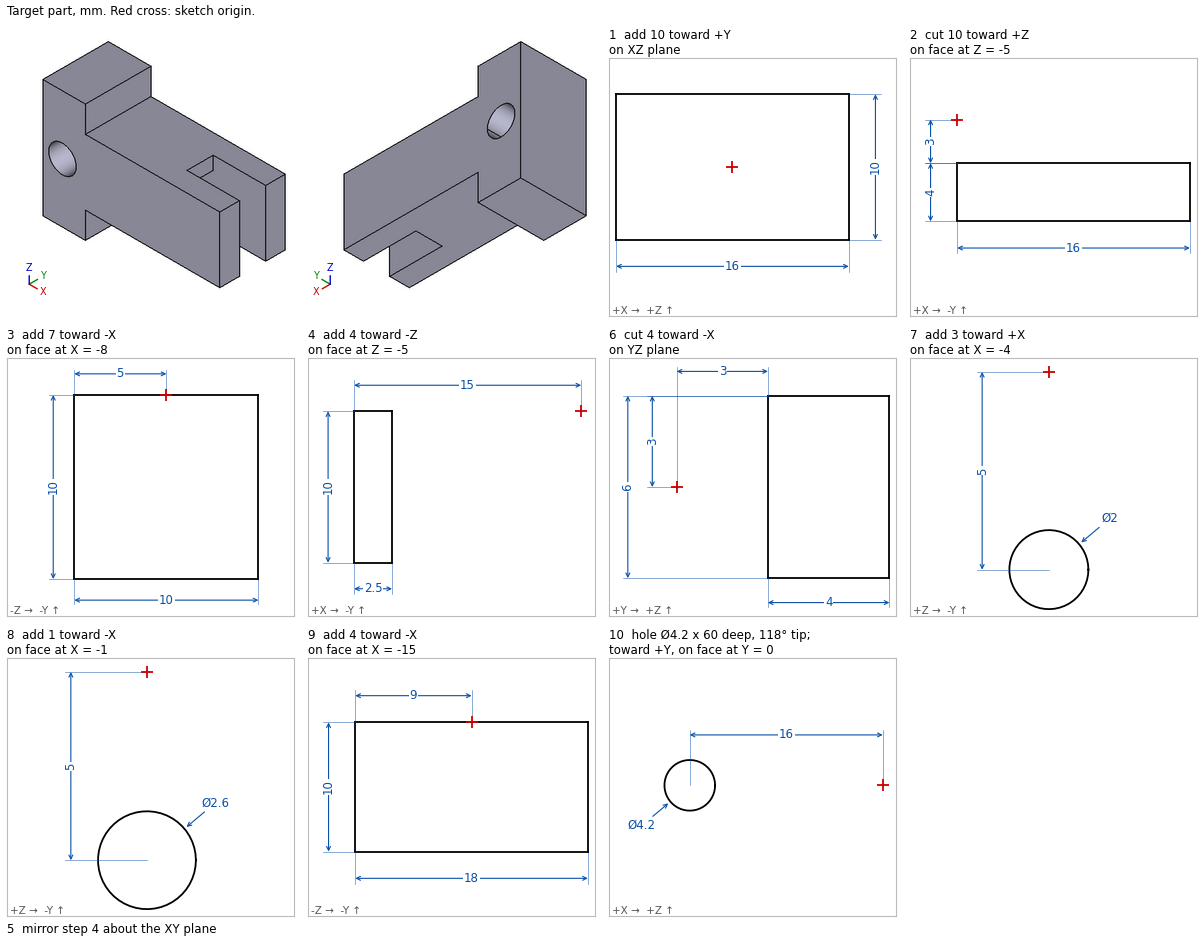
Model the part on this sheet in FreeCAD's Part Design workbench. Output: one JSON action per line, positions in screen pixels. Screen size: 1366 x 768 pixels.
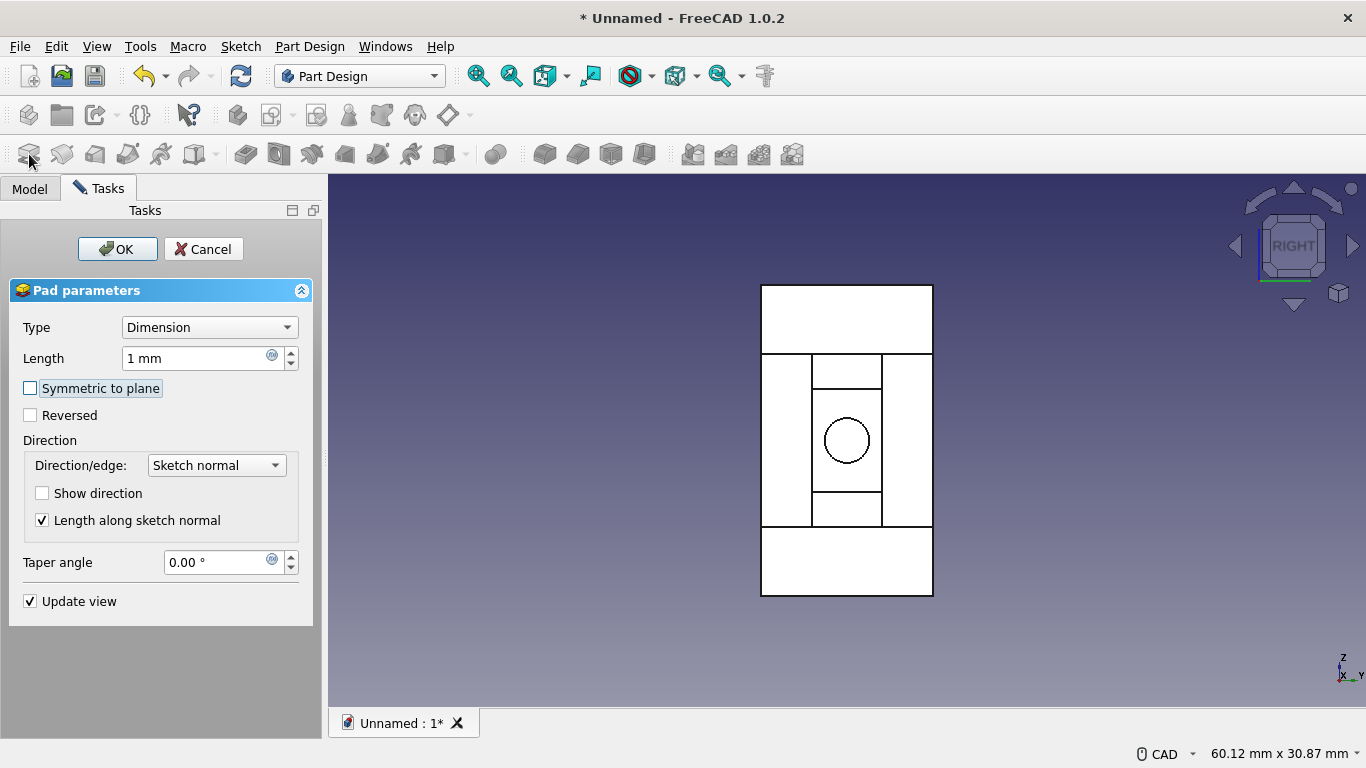
{"action": "left_click", "coordinate": [31, 415]}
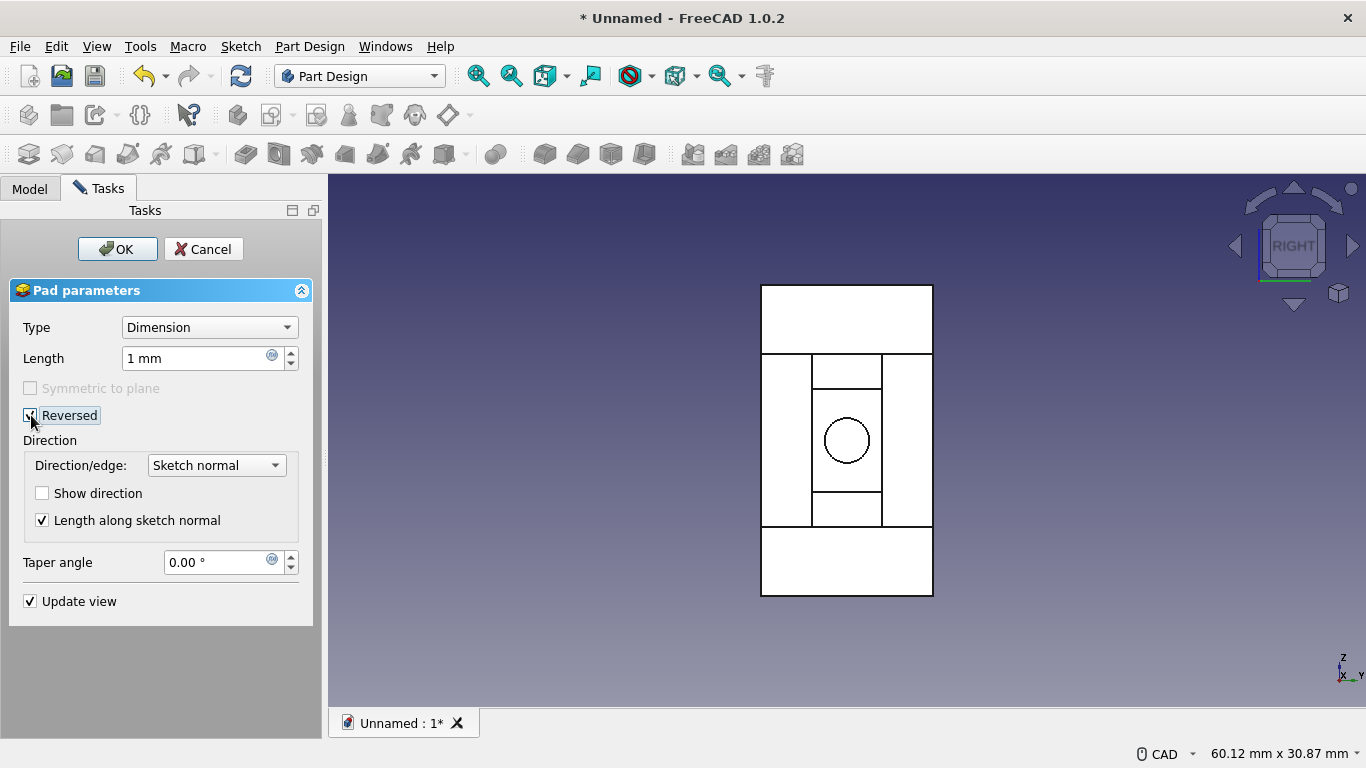
{"action": "left_click", "coordinate": [118, 249]}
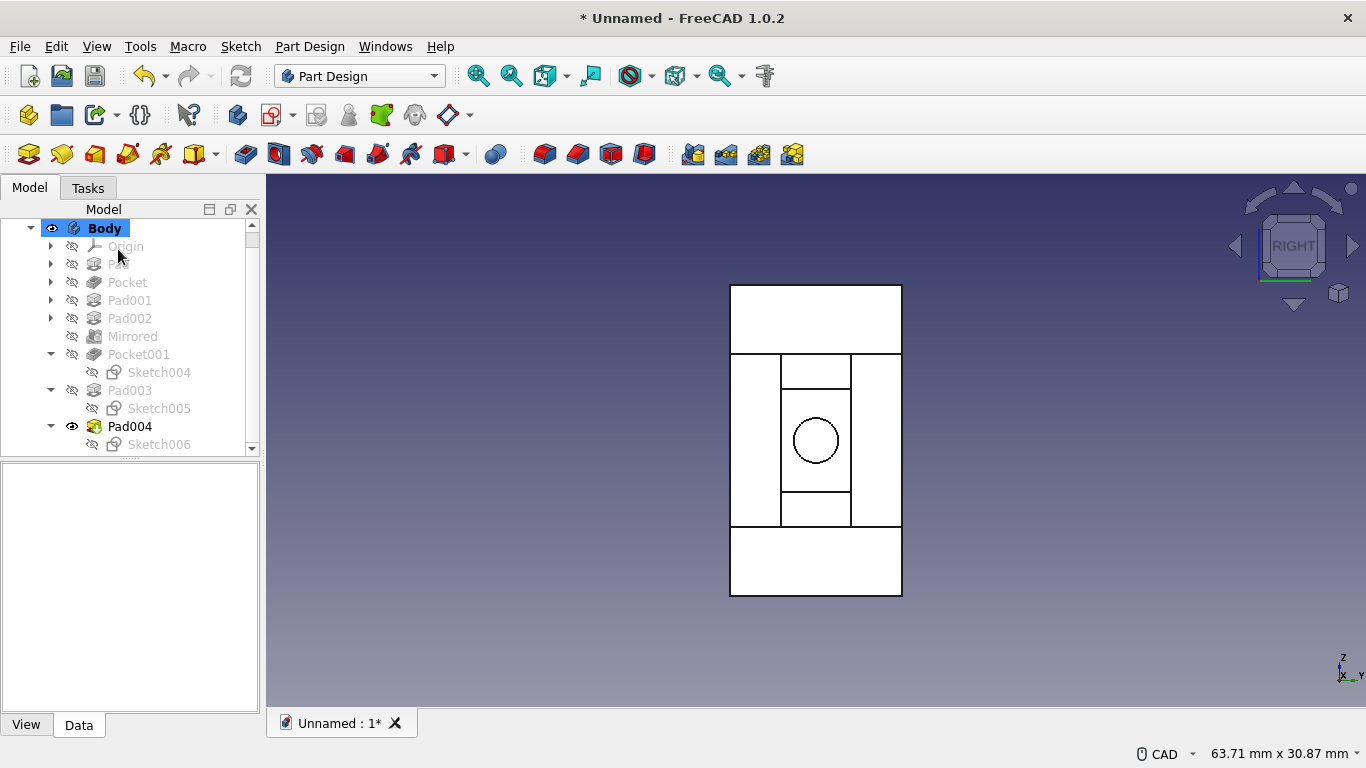
{"action": "key", "text": "6"}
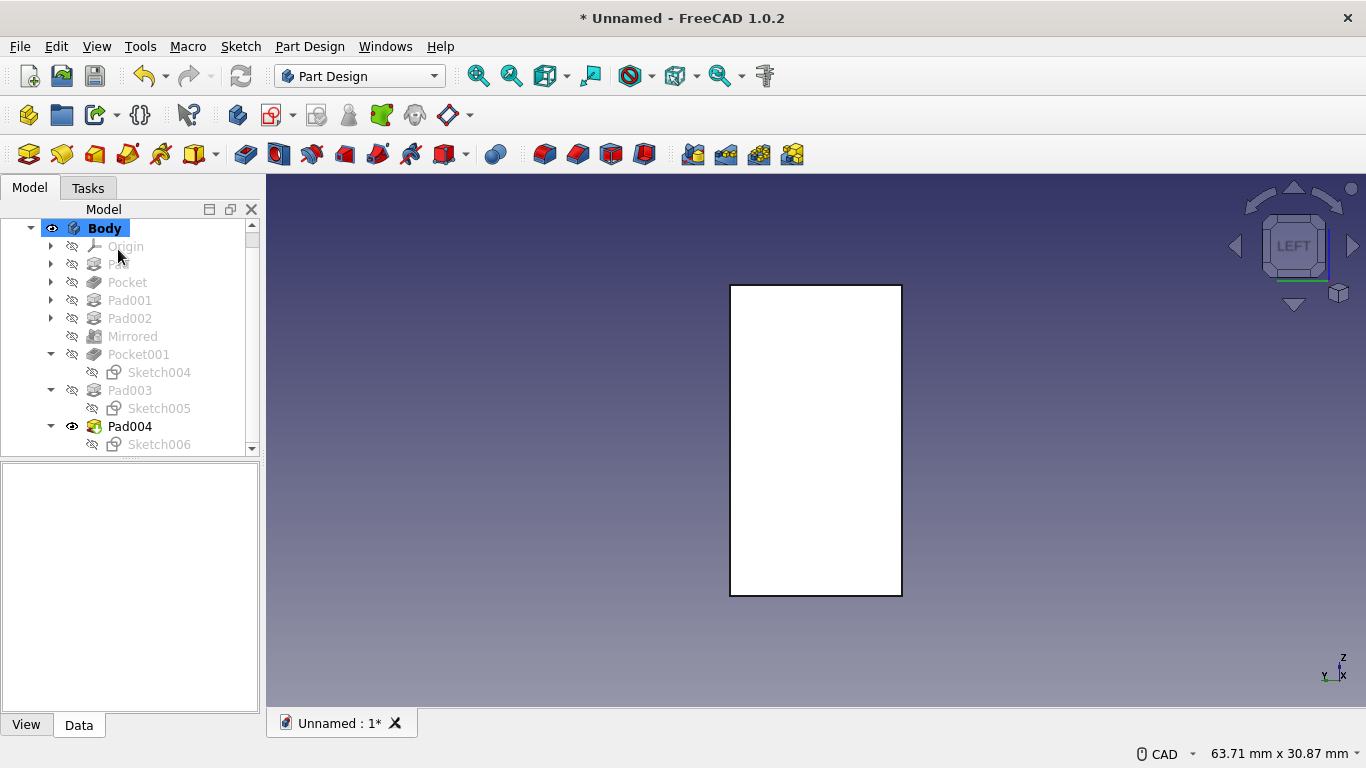
{"action": "left_click", "coordinate": [816, 395]}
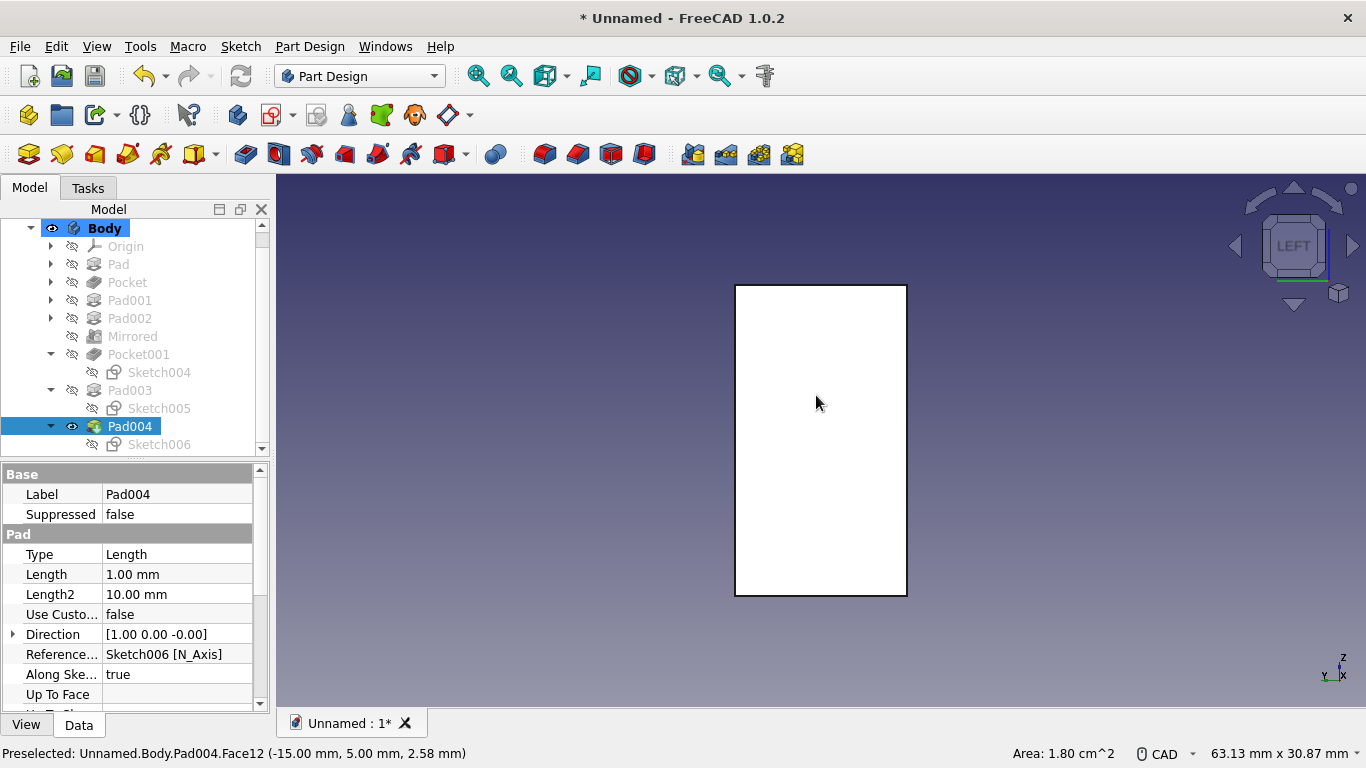
{"action": "left_click", "coordinate": [270, 116]}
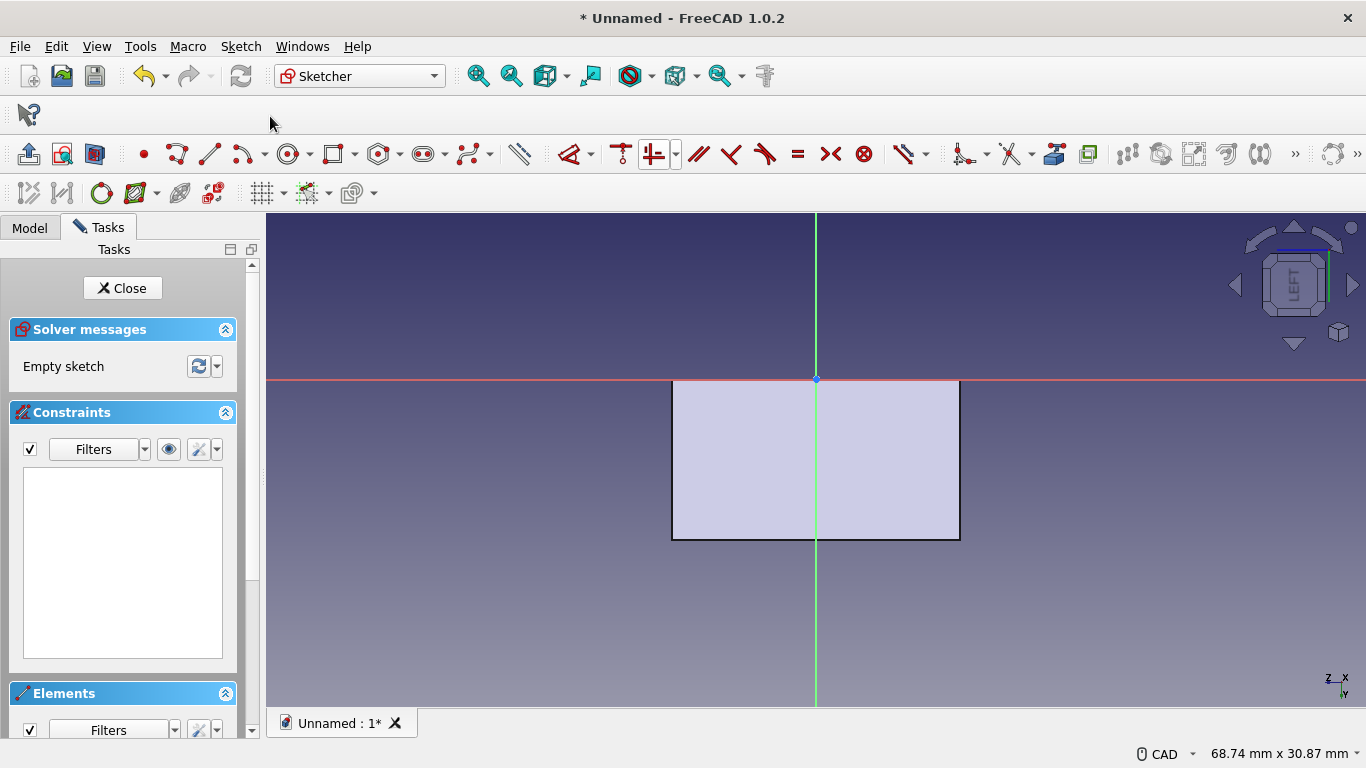
{"action": "scroll", "coordinate": [899, 460], "scroll_direction": "up", "scroll_amount": 3}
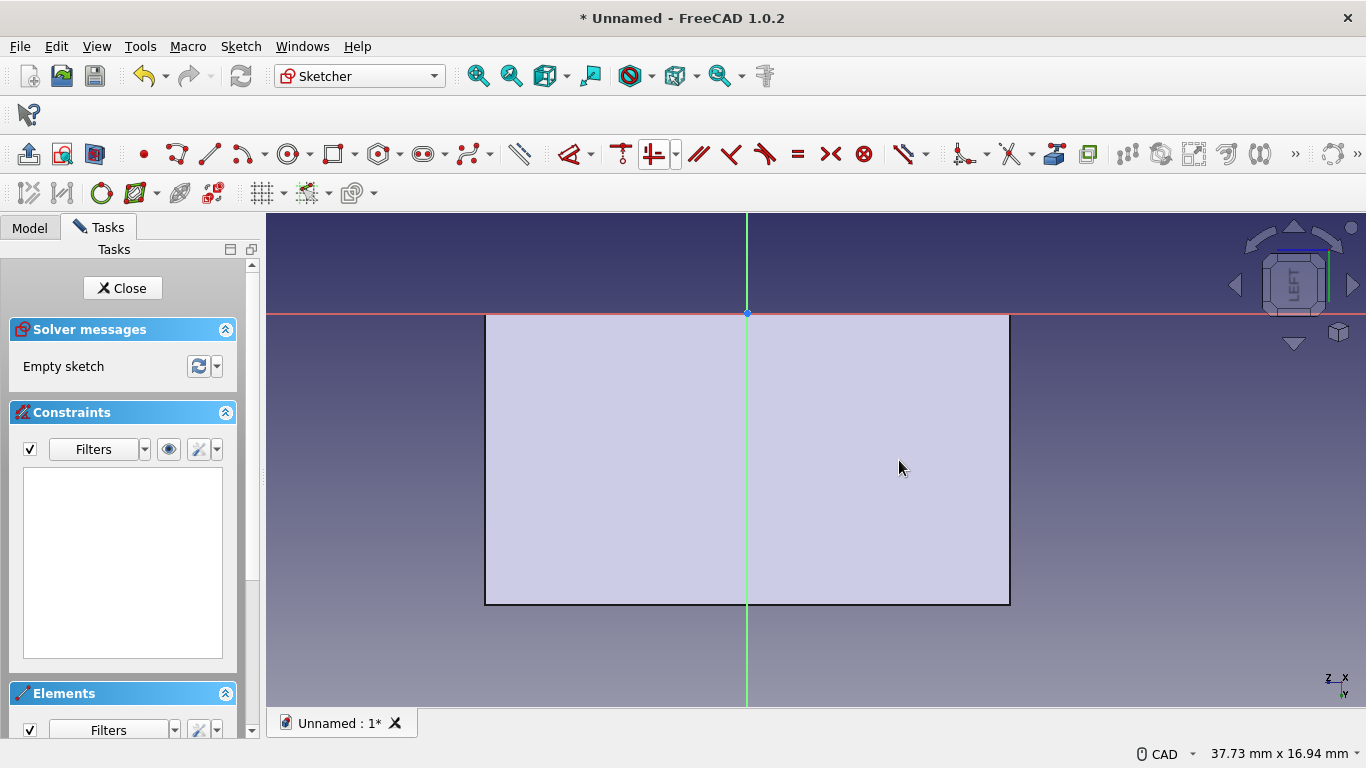
{"action": "left_click", "coordinate": [332, 154]}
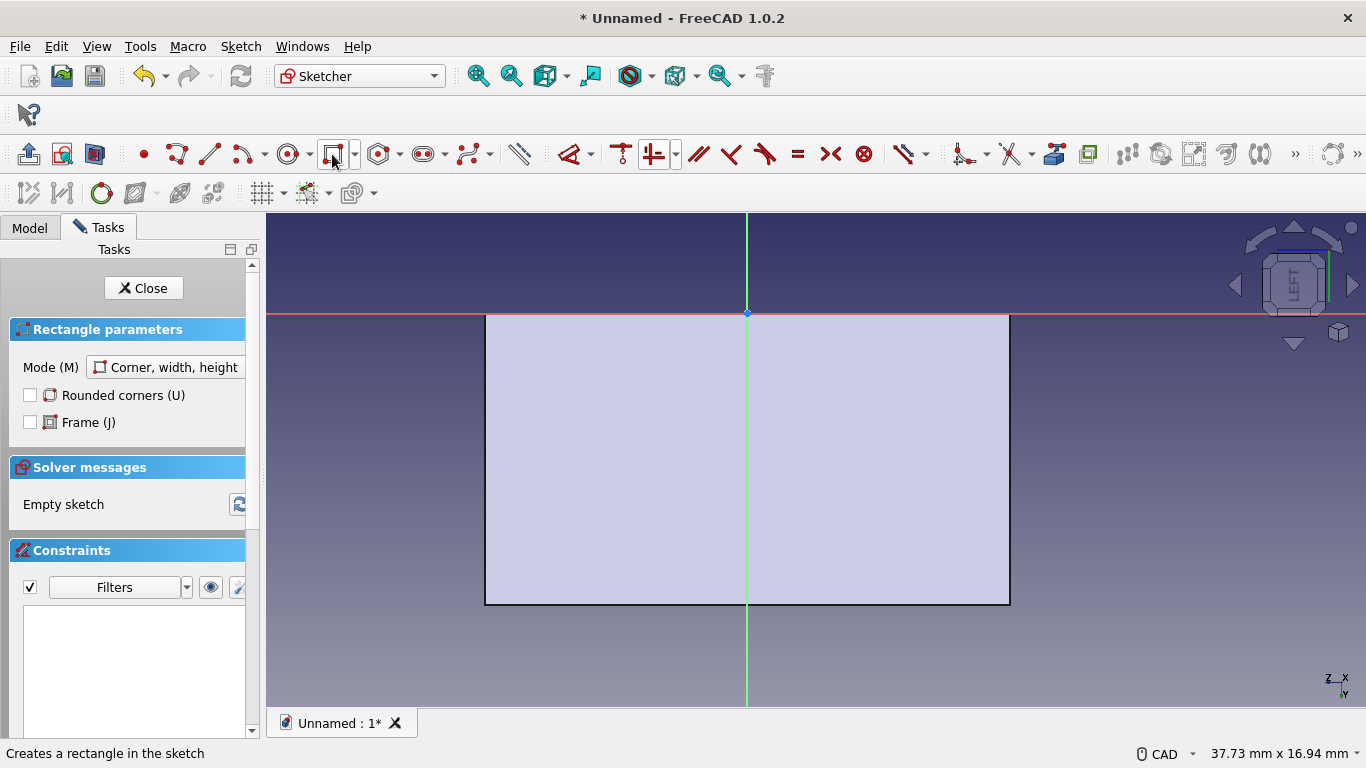
{"action": "left_click", "coordinate": [485, 314]}
{"action": "left_click", "coordinate": [1010, 605]}
{"action": "key", "text": "Escape"}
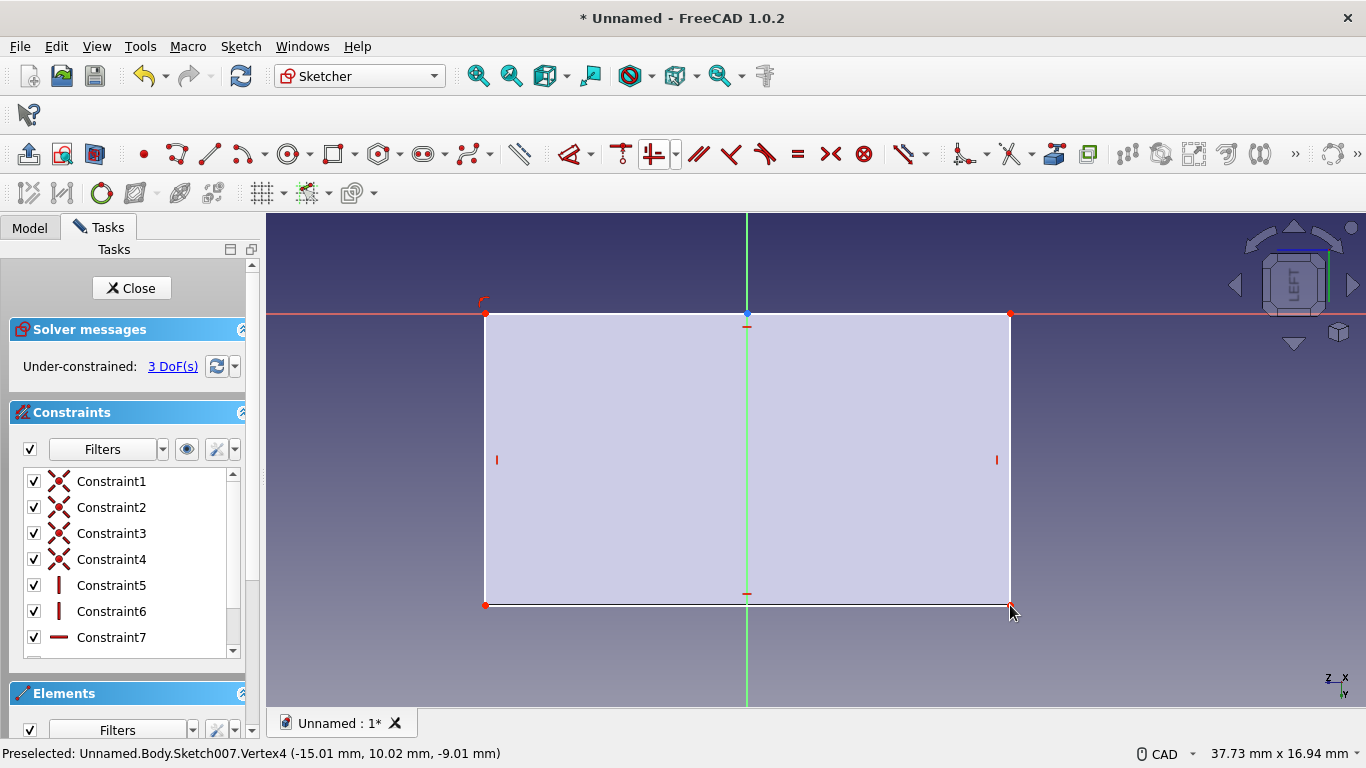
{"action": "left_click", "coordinate": [568, 154]}